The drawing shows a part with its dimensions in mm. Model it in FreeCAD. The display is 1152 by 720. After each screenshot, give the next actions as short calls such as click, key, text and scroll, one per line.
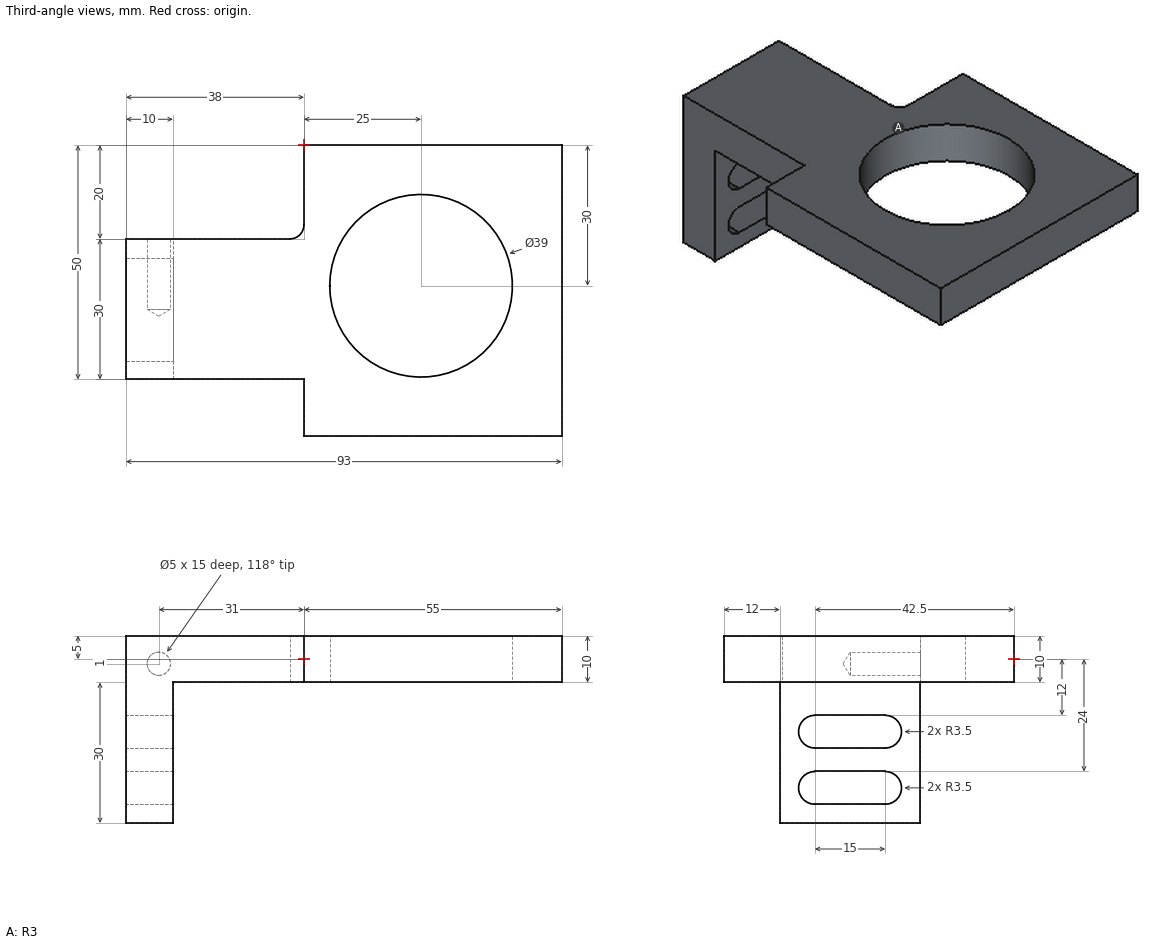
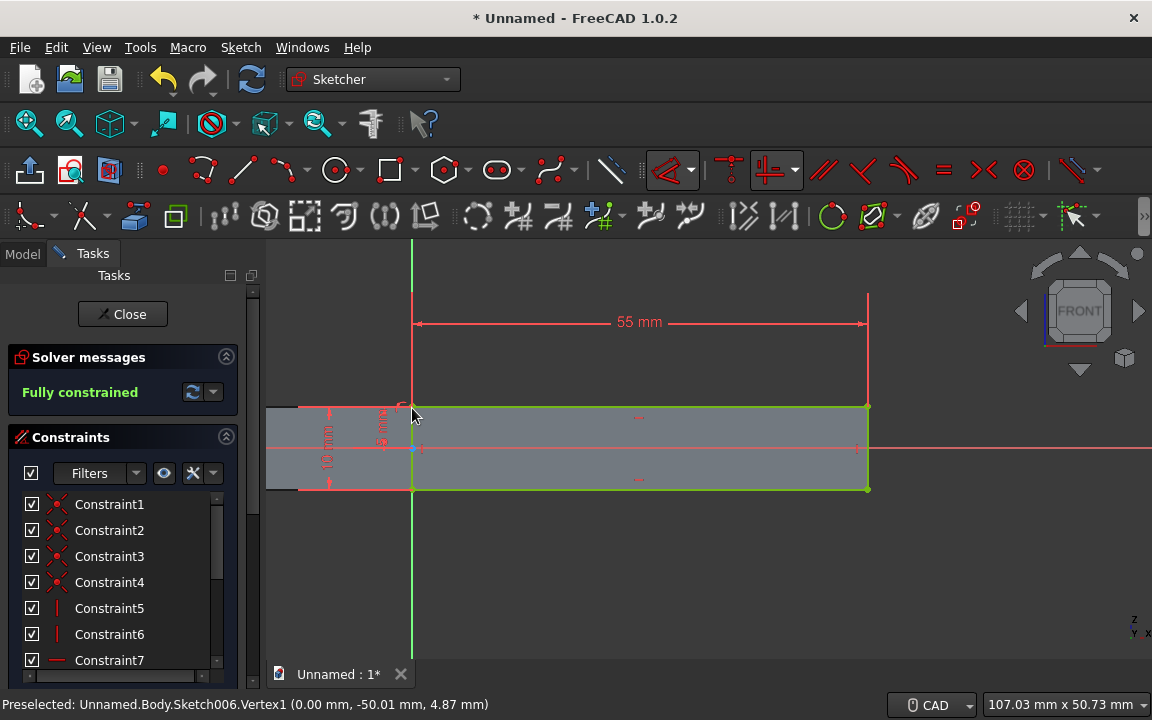
click(123, 314)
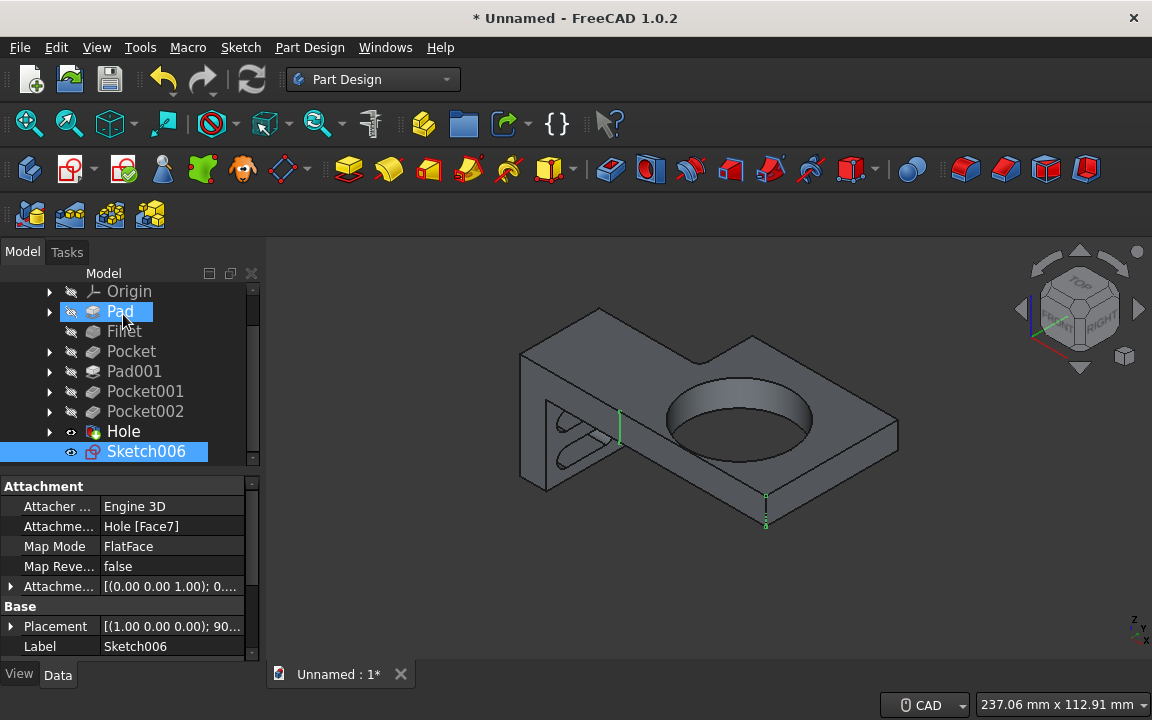
click(350, 170)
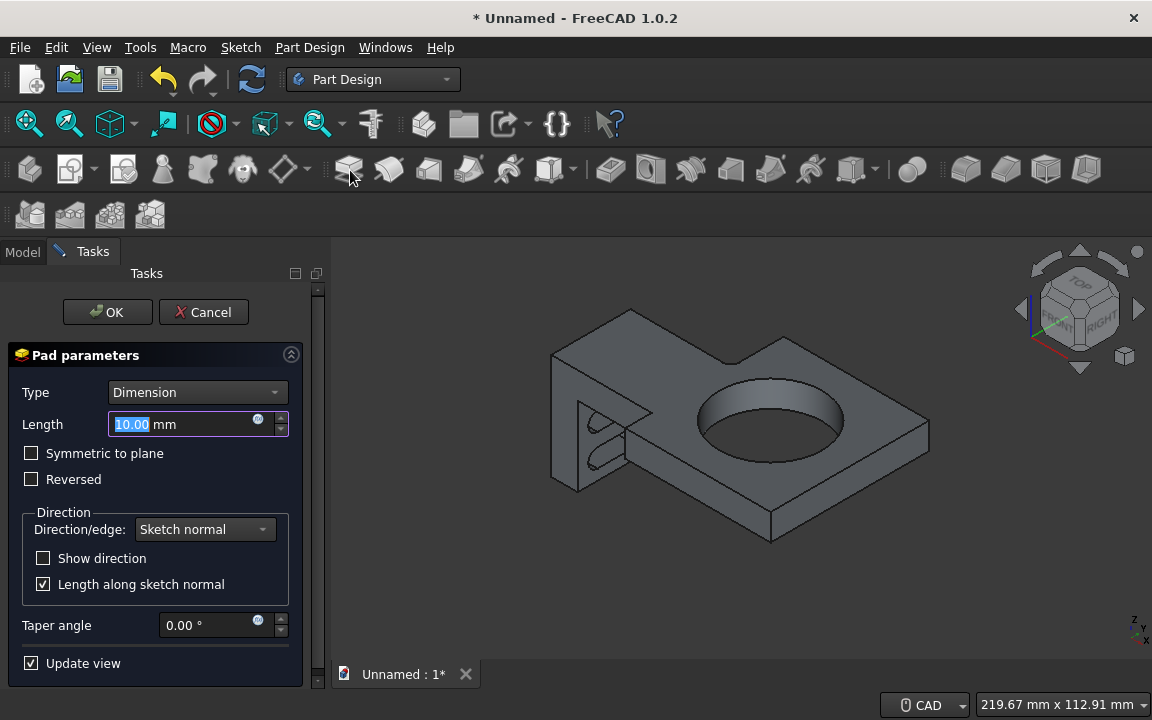
text(12)
key(Tab)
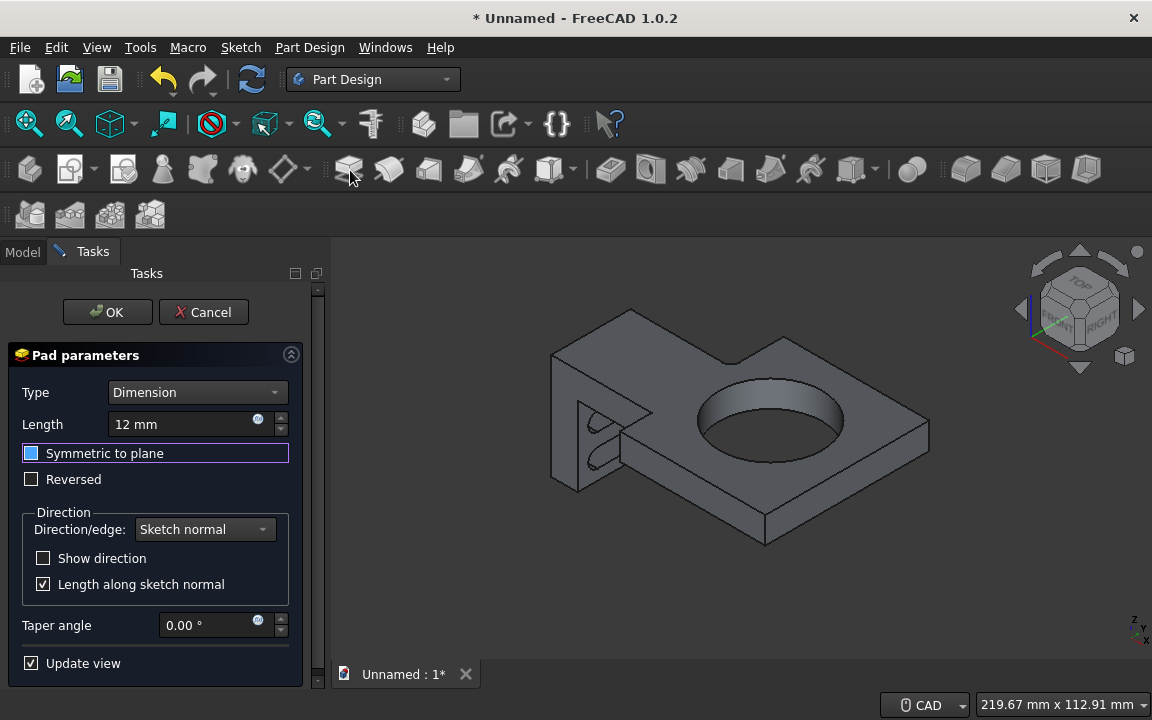
click(108, 312)